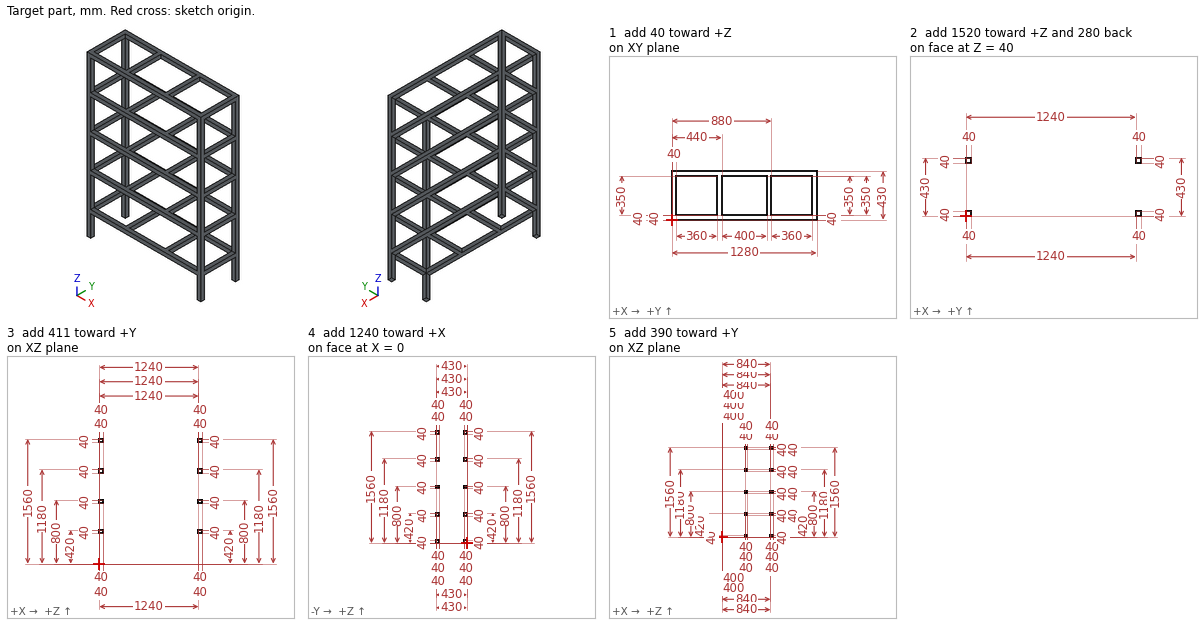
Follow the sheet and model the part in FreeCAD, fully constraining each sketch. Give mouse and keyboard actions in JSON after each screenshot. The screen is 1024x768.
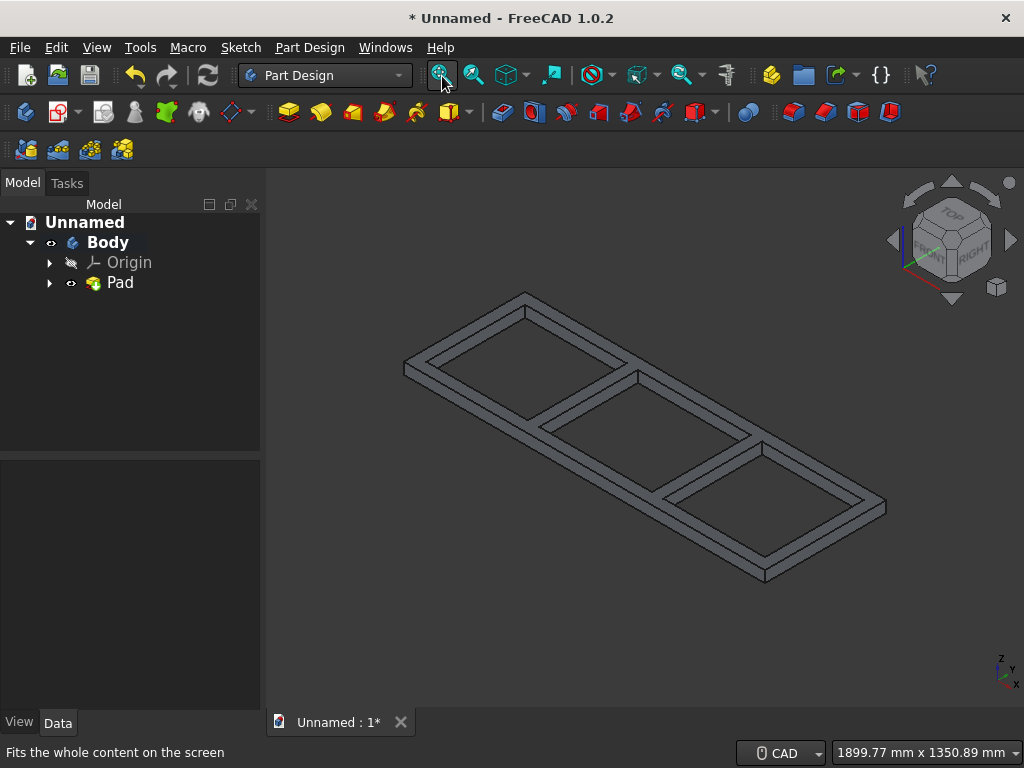
{"action": "scroll", "coordinate": [852, 489], "scroll_direction": "up", "scroll_amount": 6}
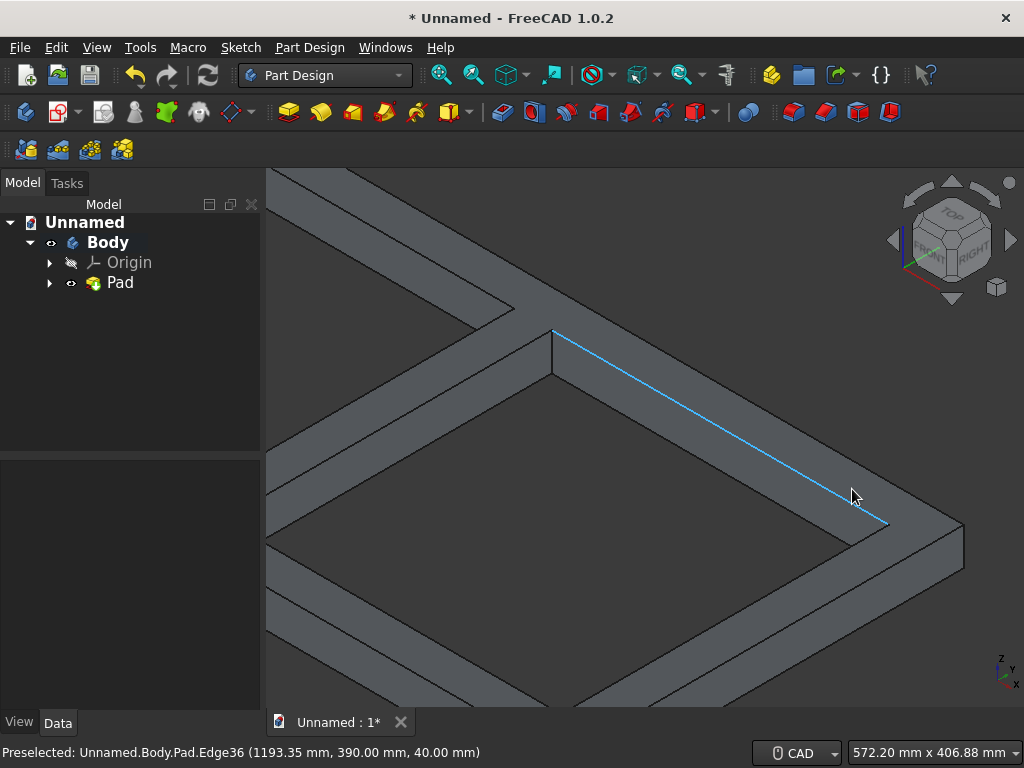
{"action": "left_click", "coordinate": [333, 591]}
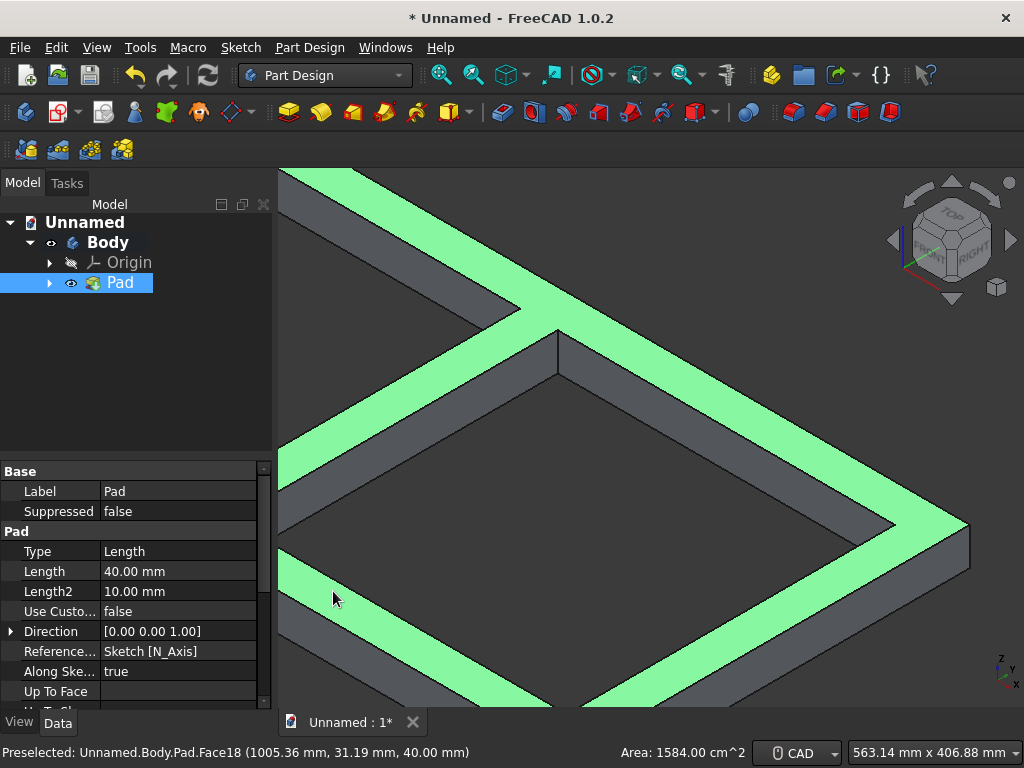
{"action": "left_click", "coordinate": [58, 112]}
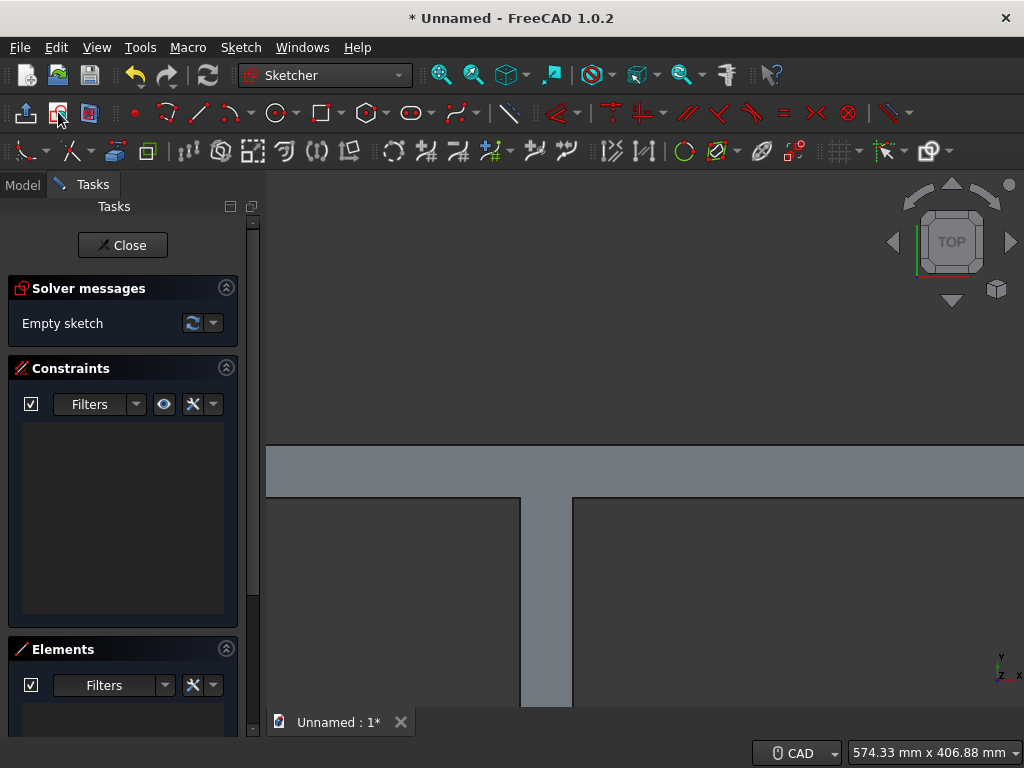
{"action": "scroll", "coordinate": [681, 343], "scroll_direction": "down", "scroll_amount": 7}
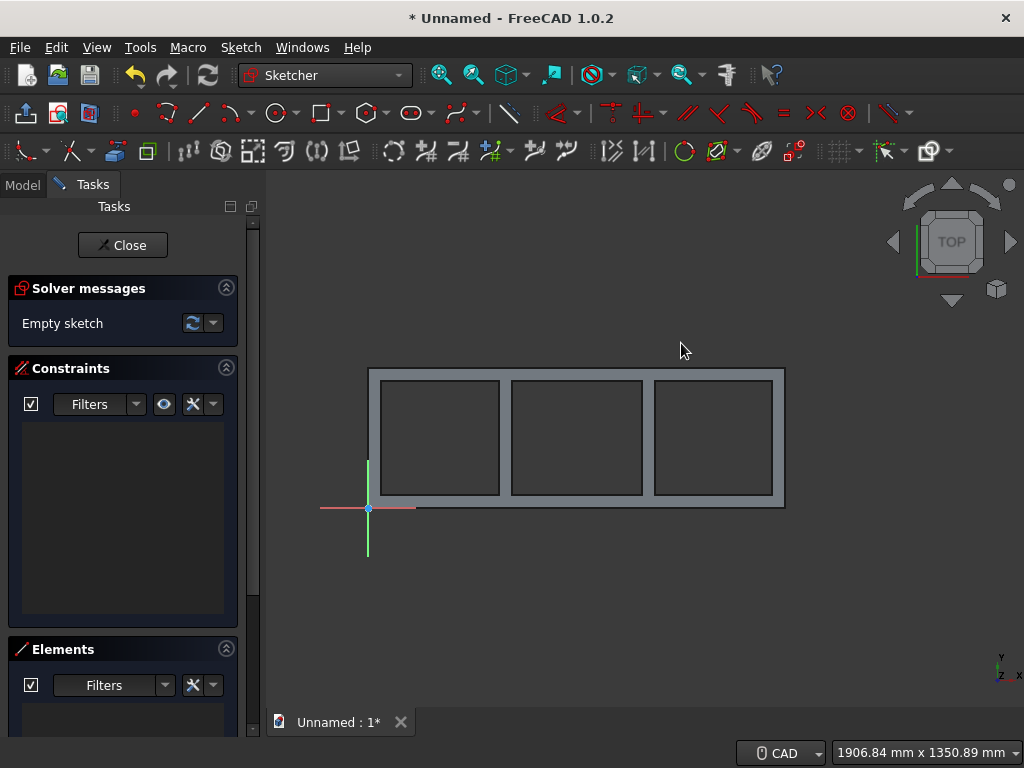
{"action": "left_click", "coordinate": [322, 114]}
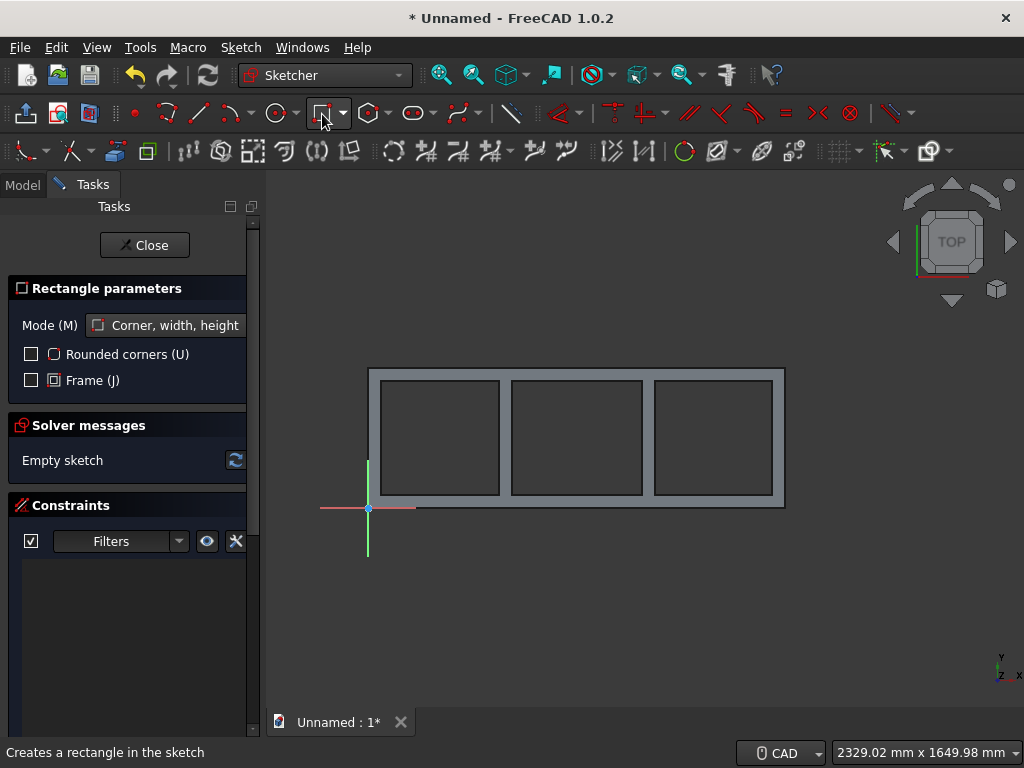
{"action": "left_click", "coordinate": [368, 368]}
{"action": "mouse_move", "coordinate": [381, 381]}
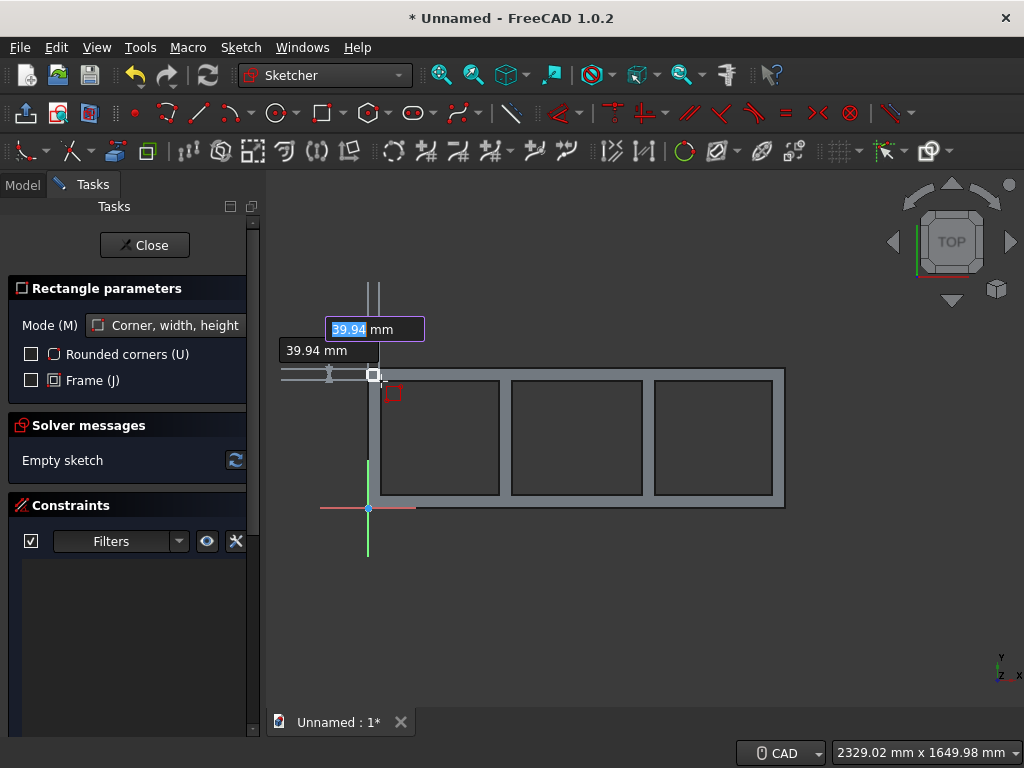
{"action": "type", "text": "40"}
{"action": "key", "text": "Tab"}
{"action": "type", "text": "40"}
{"action": "key", "text": "Return"}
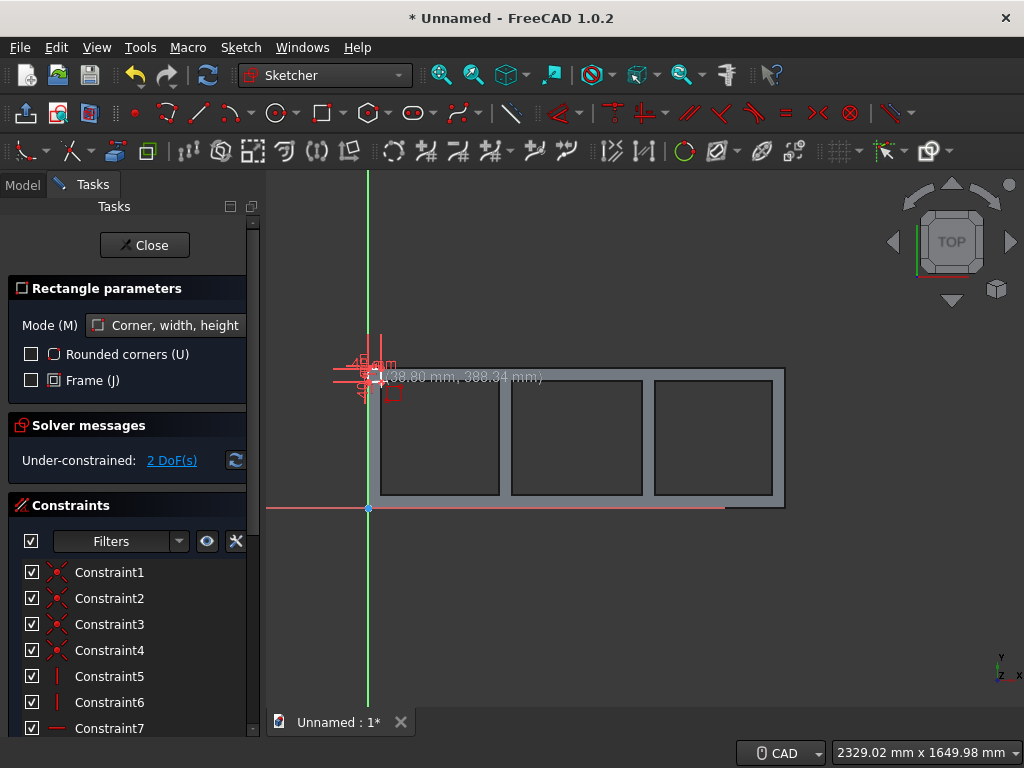
{"action": "left_click", "coordinate": [368, 508]}
{"action": "mouse_move", "coordinate": [381, 495]}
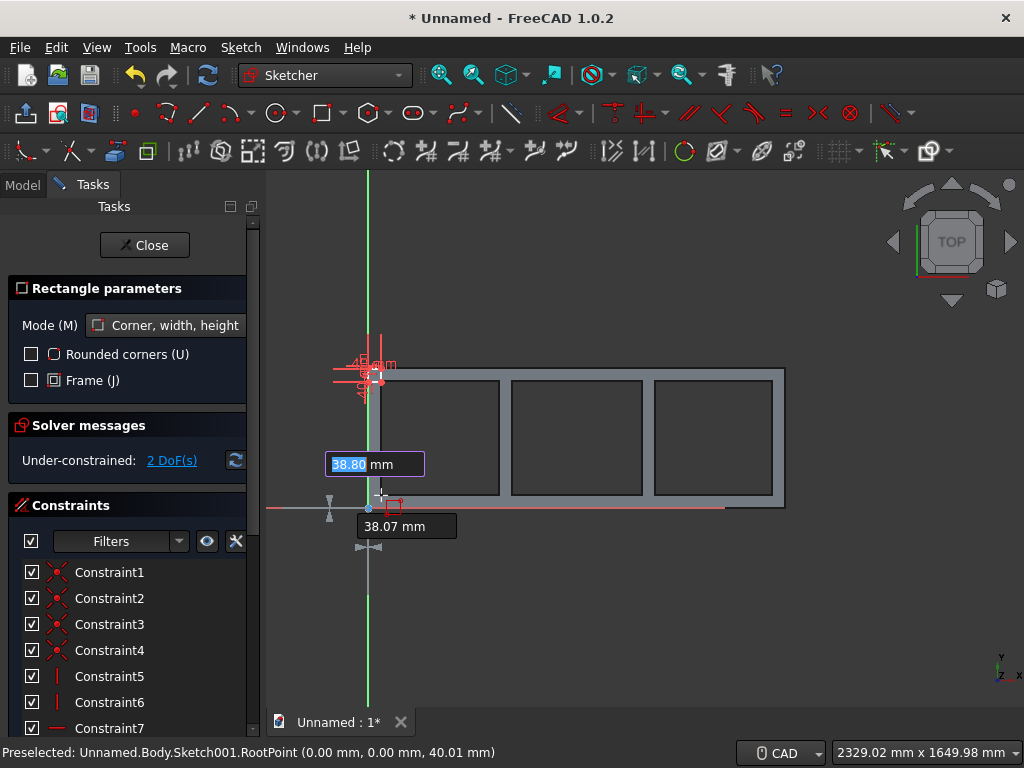
{"action": "type", "text": "40"}
{"action": "key", "text": "Tab"}
{"action": "type", "text": "40"}
{"action": "key", "text": "Return"}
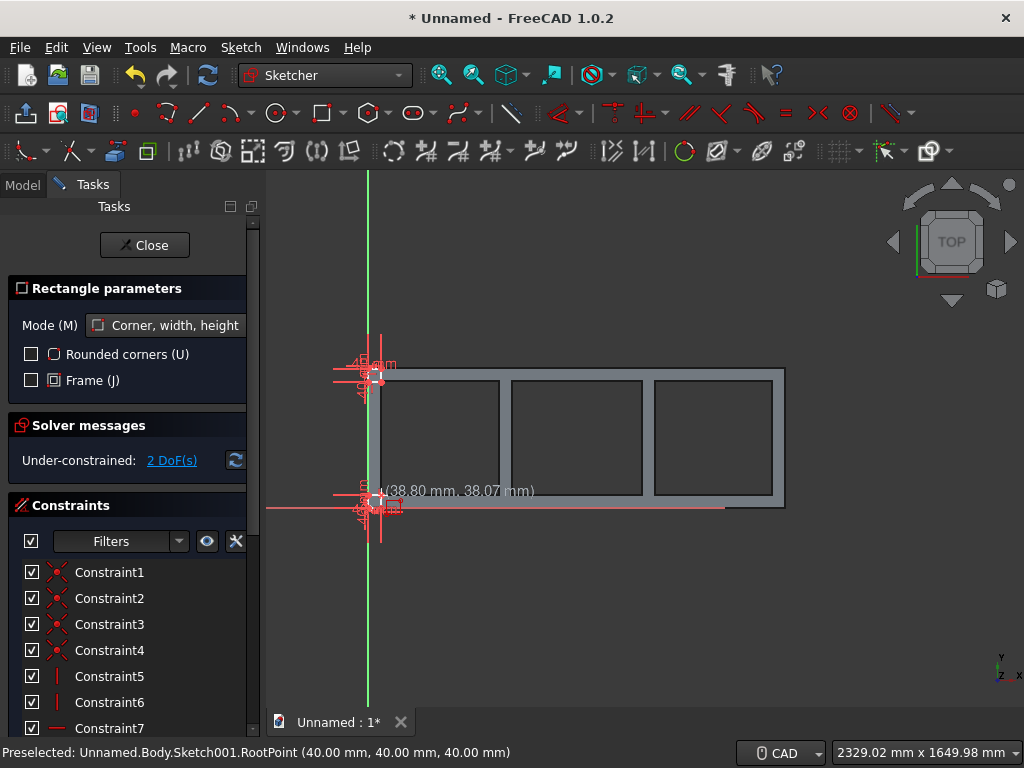
{"action": "left_click", "coordinate": [772, 495]}
{"action": "left_click", "coordinate": [785, 508]}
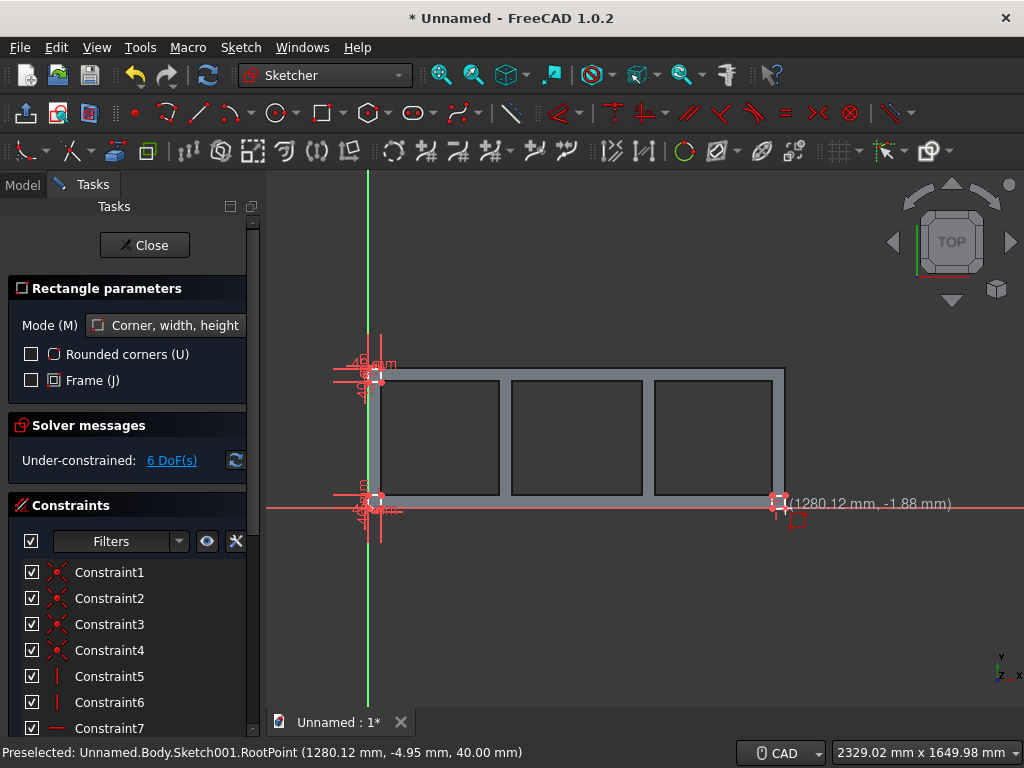
{"action": "left_click", "coordinate": [772, 368]}
{"action": "mouse_move", "coordinate": [785, 381]}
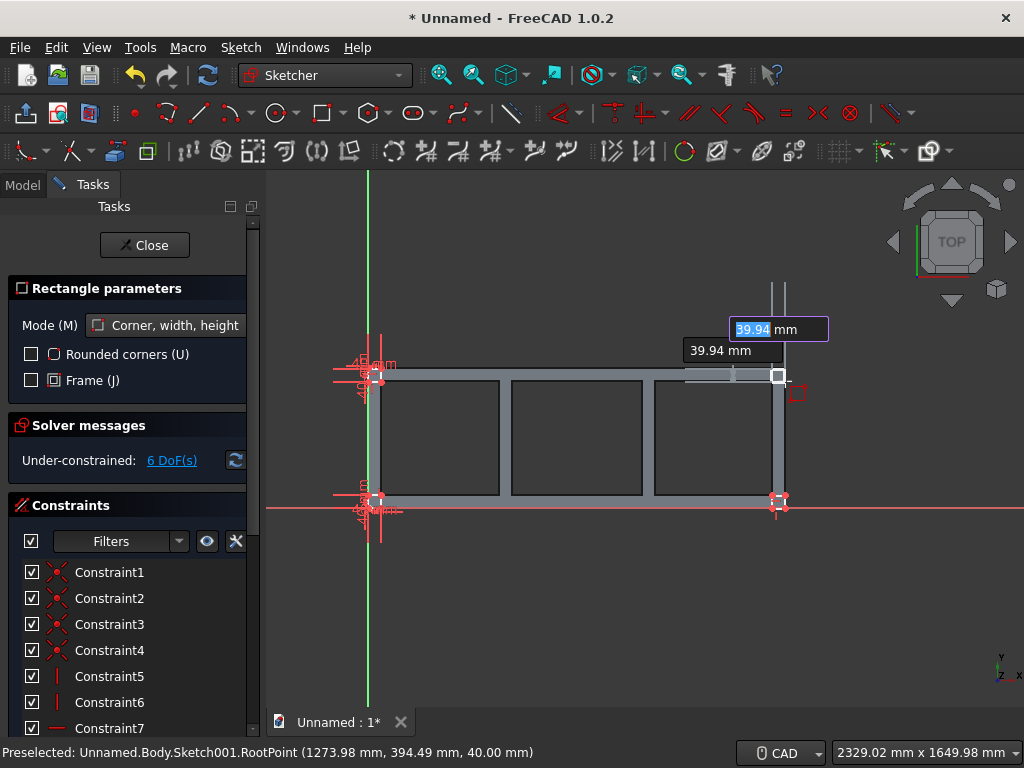
{"action": "type", "text": "40"}
{"action": "key", "text": "Tab"}
{"action": "type", "text": "40"}
{"action": "key", "text": "Return"}
{"action": "key", "text": "Escape"}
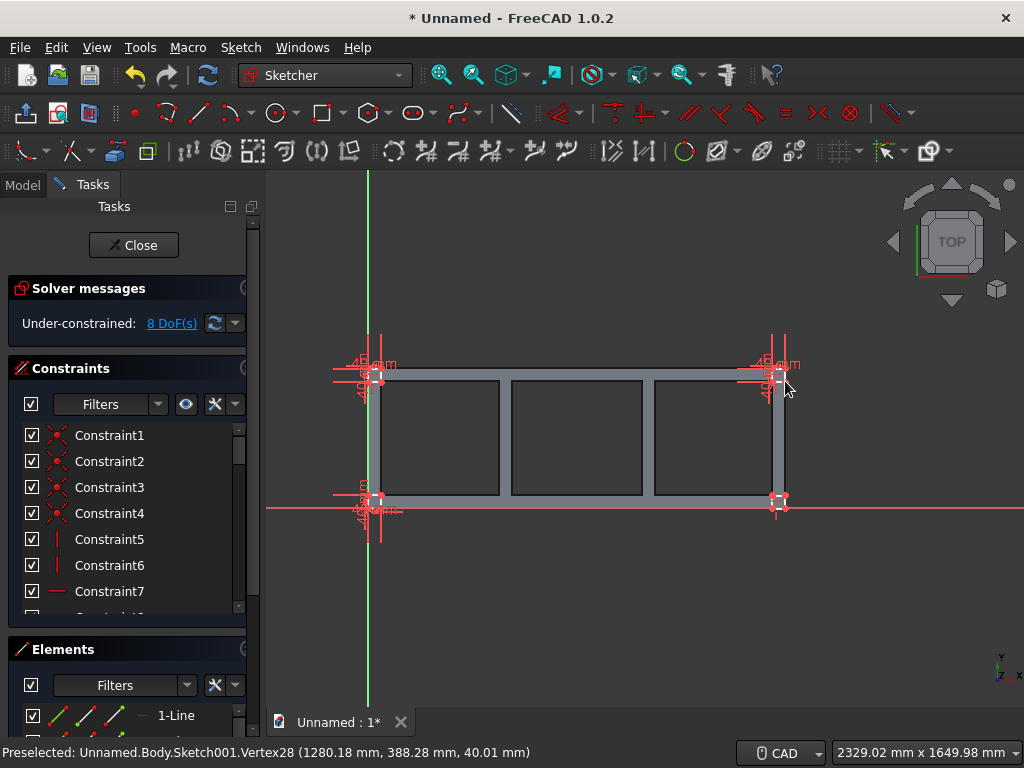
{"action": "left_click", "coordinate": [368, 369]}